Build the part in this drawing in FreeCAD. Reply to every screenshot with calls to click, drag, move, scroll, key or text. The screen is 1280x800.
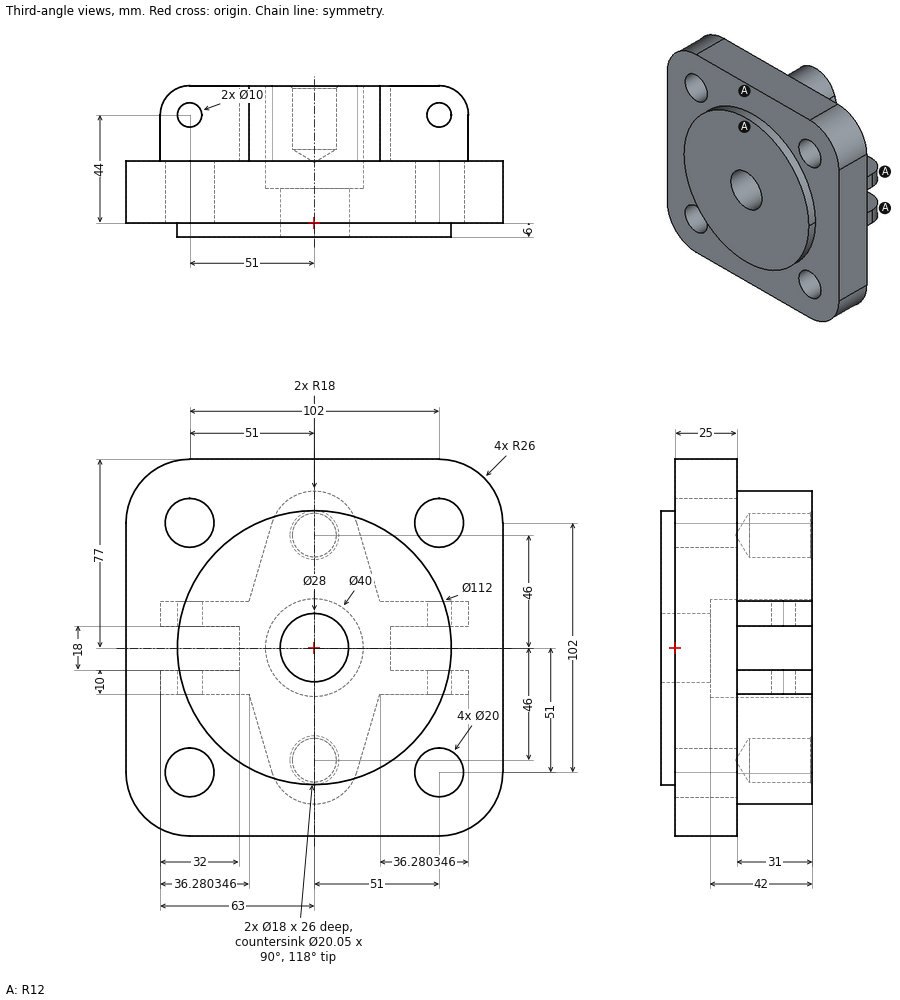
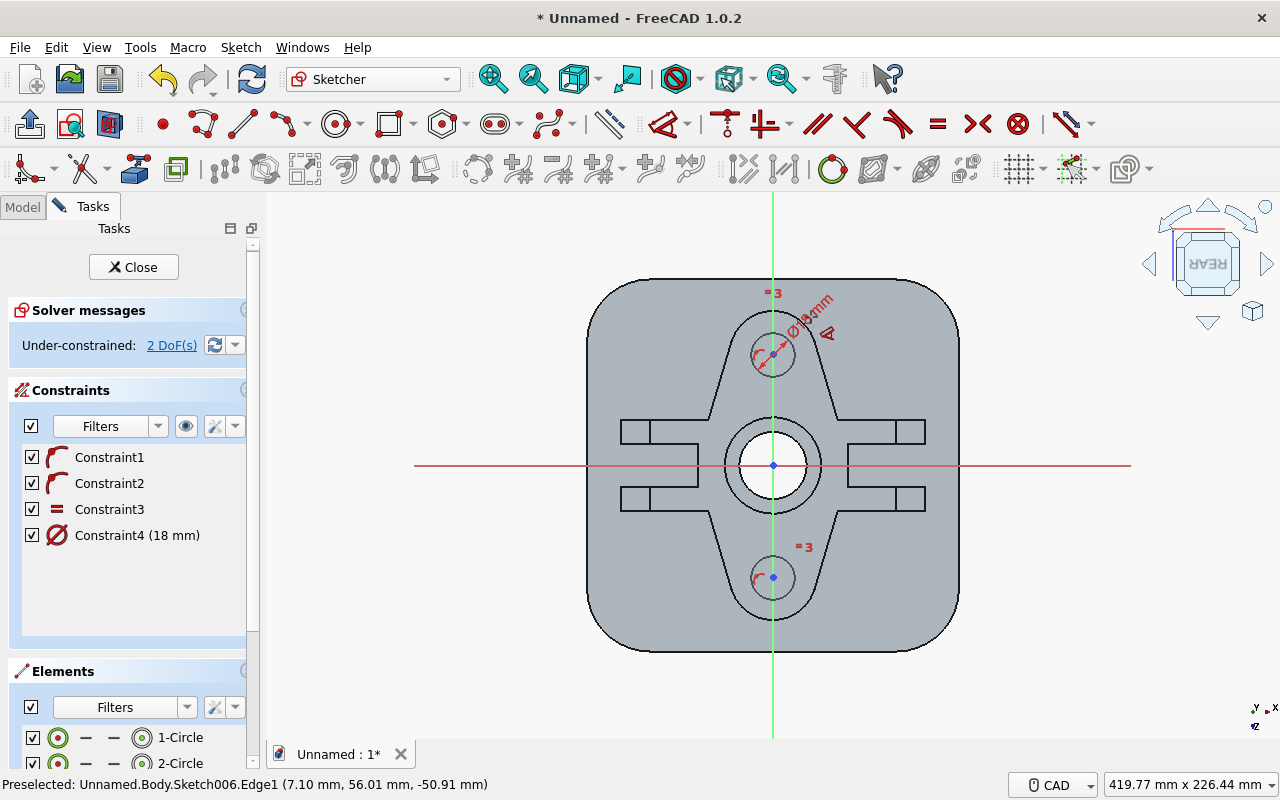
click(773, 355)
click(807, 410)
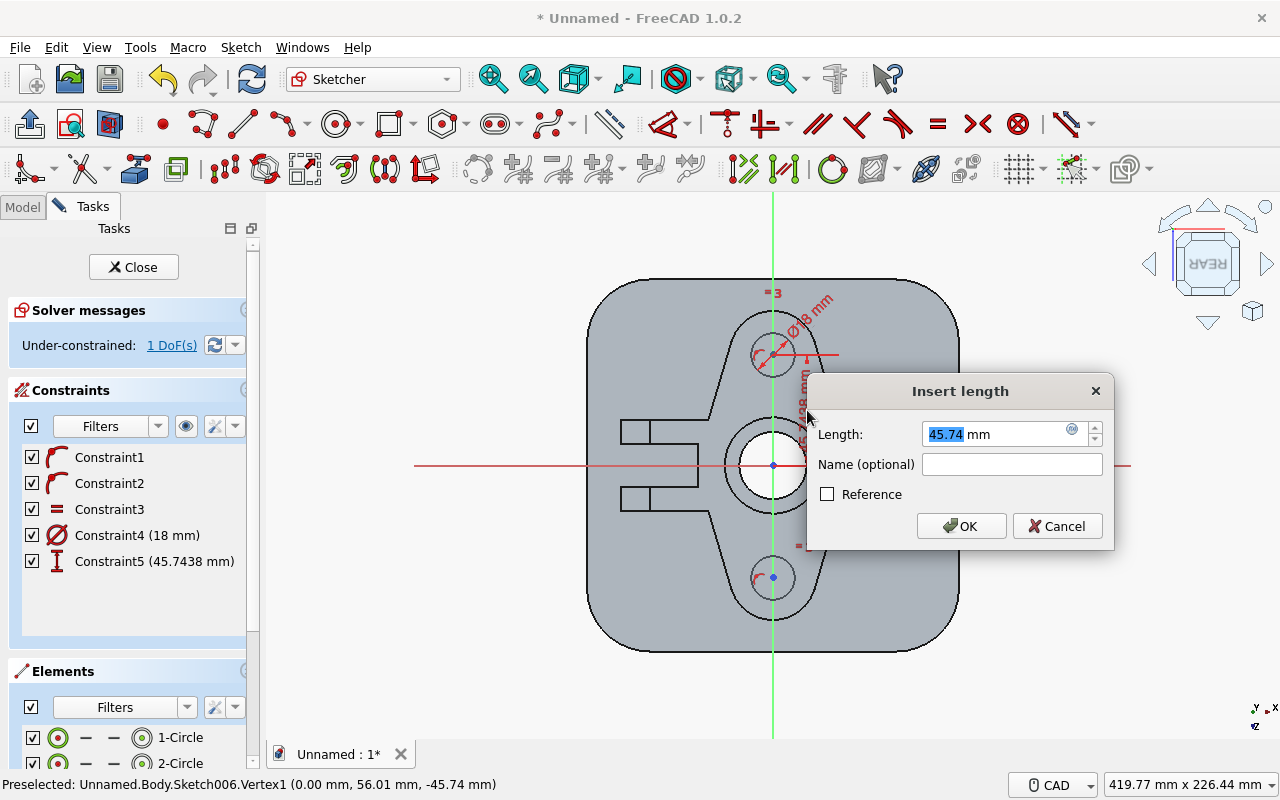
text(46)
key(Return)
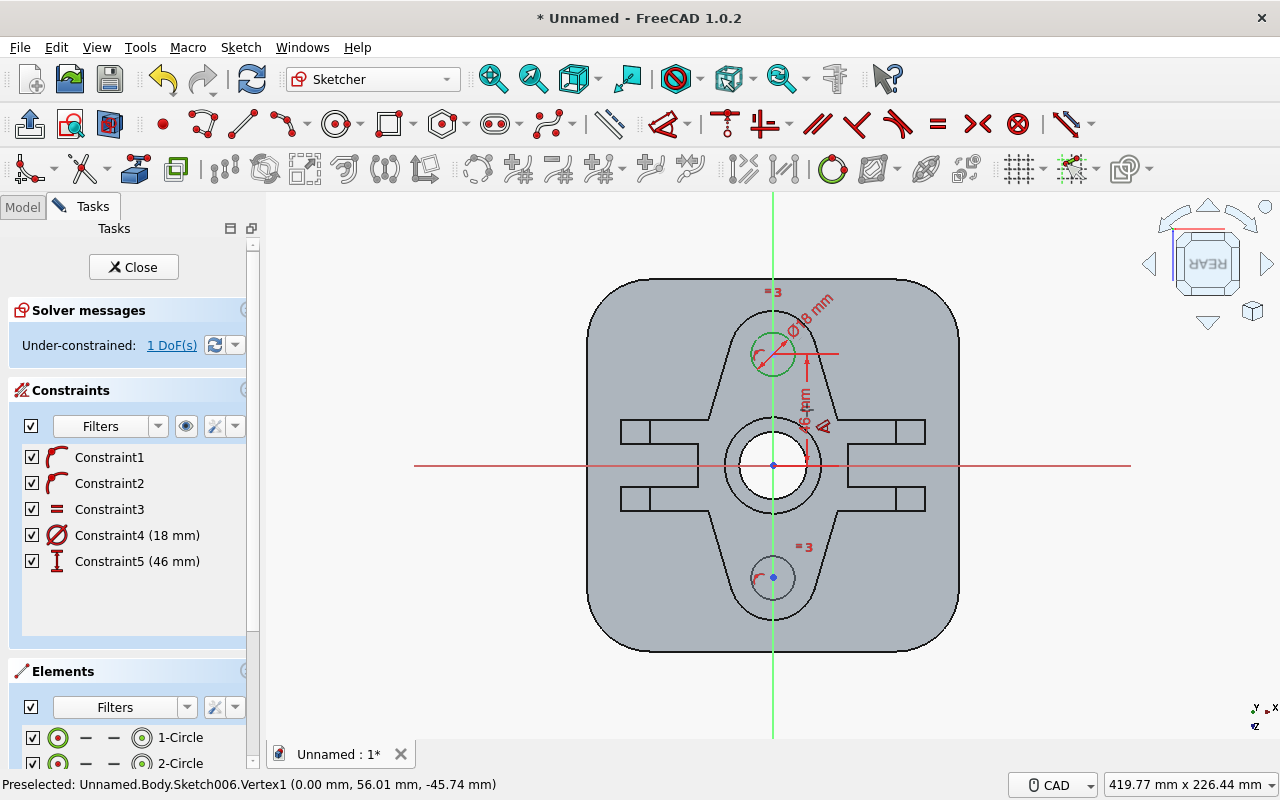
click(773, 578)
click(807, 522)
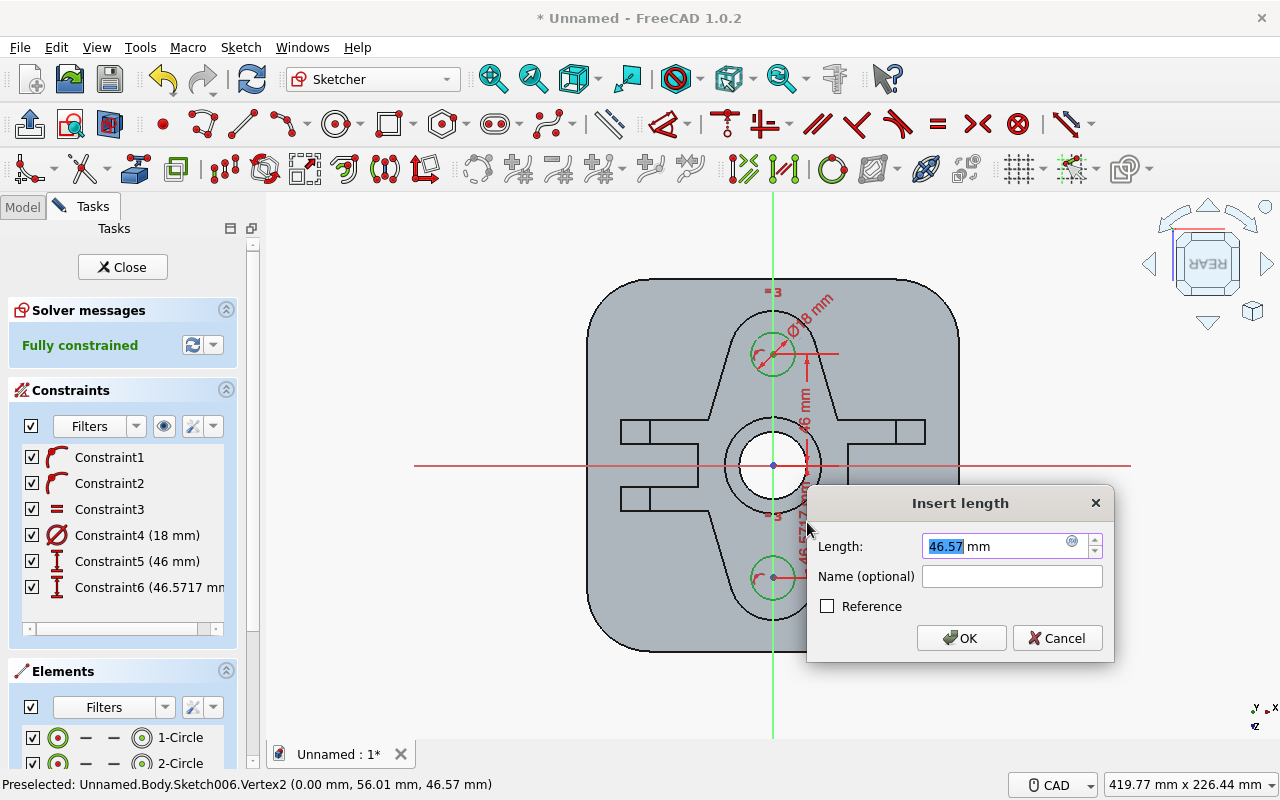
text(46)
key(Return)
key(Escape)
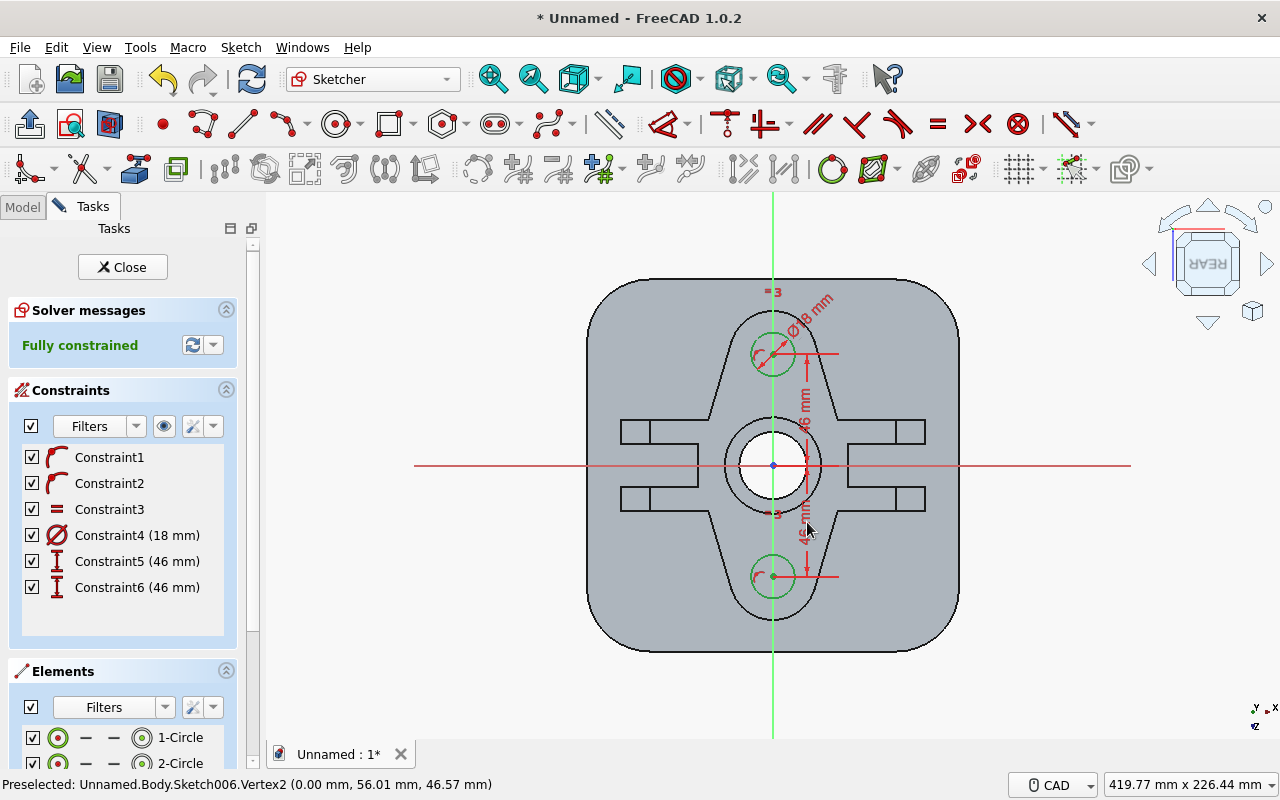
click(123, 267)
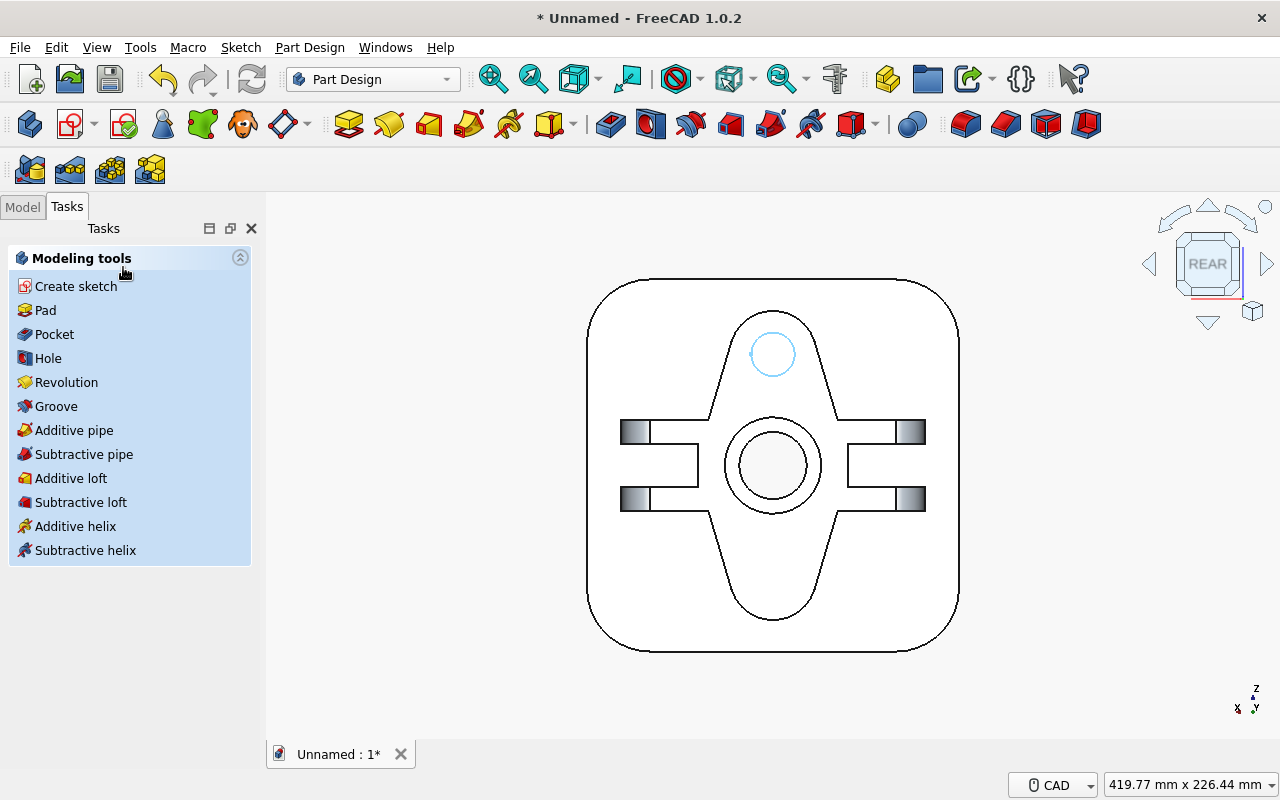
click(652, 124)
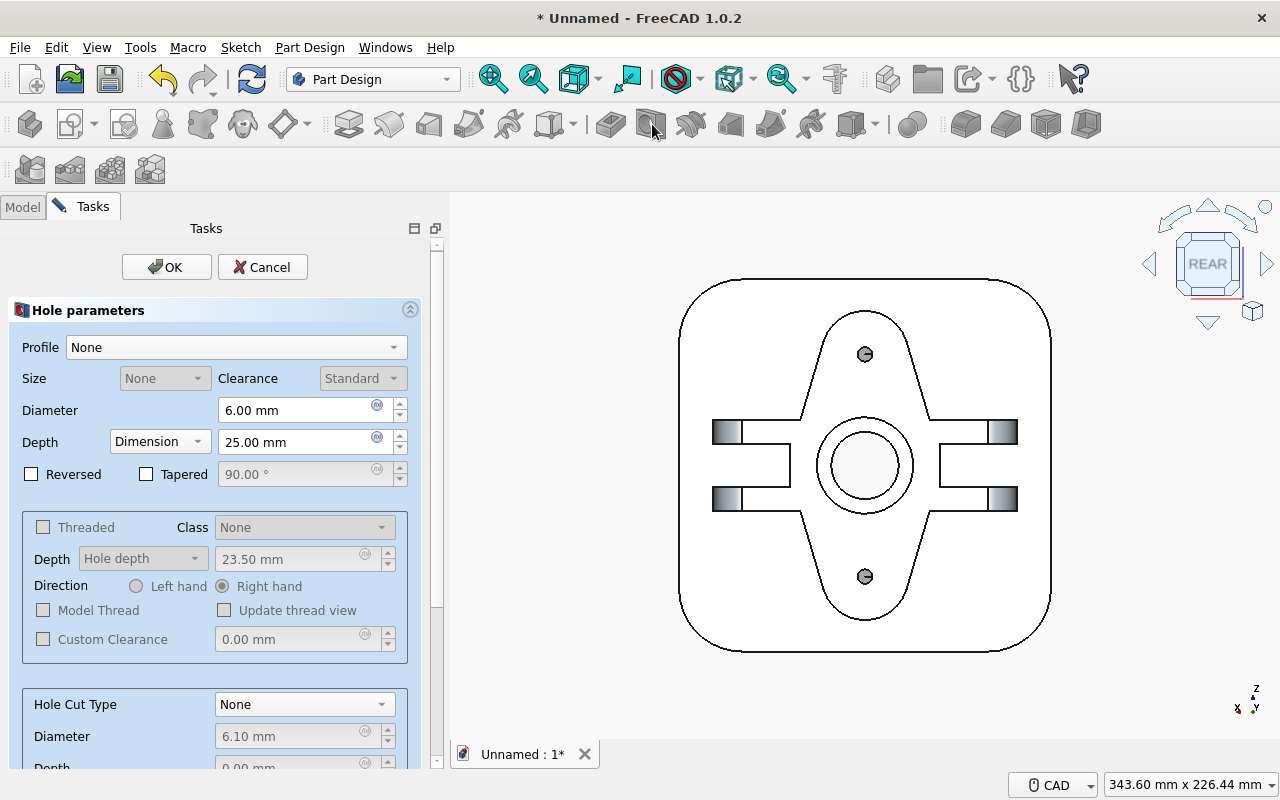
triple_click(305, 410)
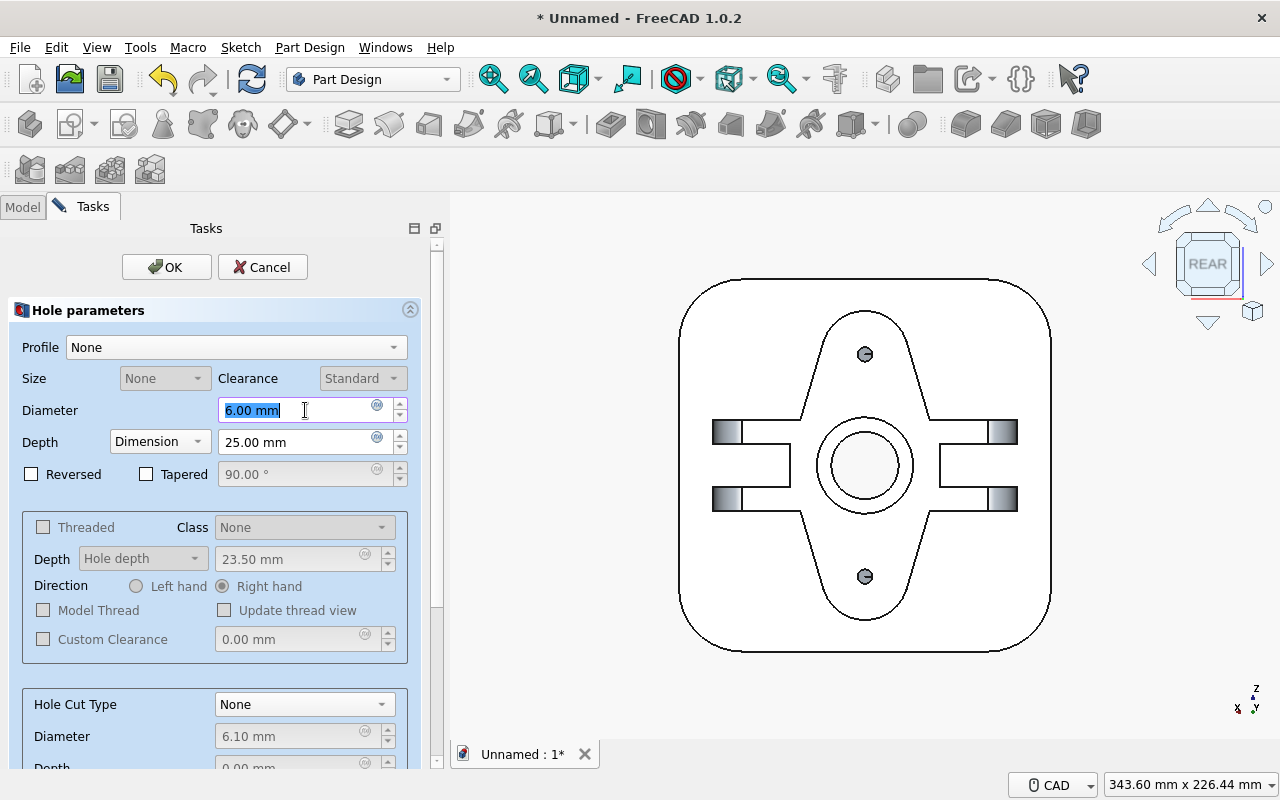
text(18)
key(Tab)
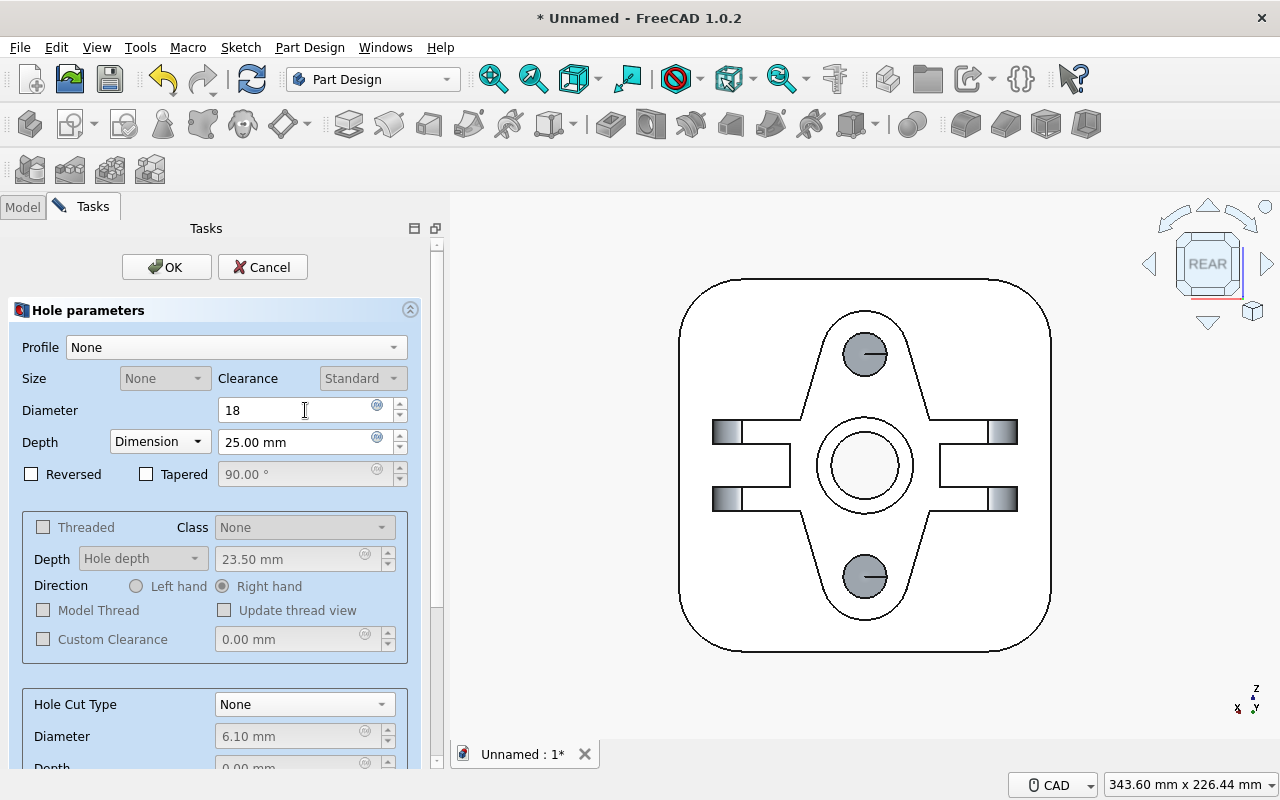
triple_click(305, 442)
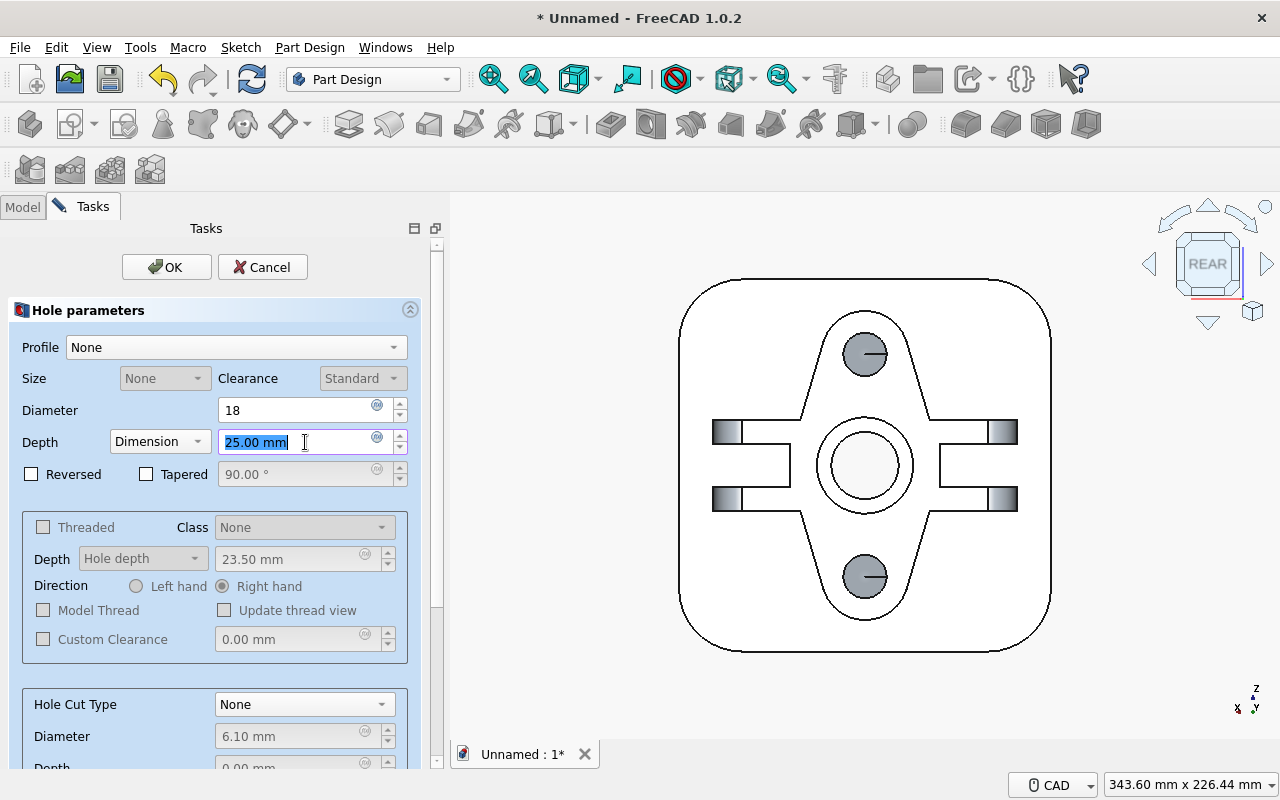
text(26)
key(Tab)